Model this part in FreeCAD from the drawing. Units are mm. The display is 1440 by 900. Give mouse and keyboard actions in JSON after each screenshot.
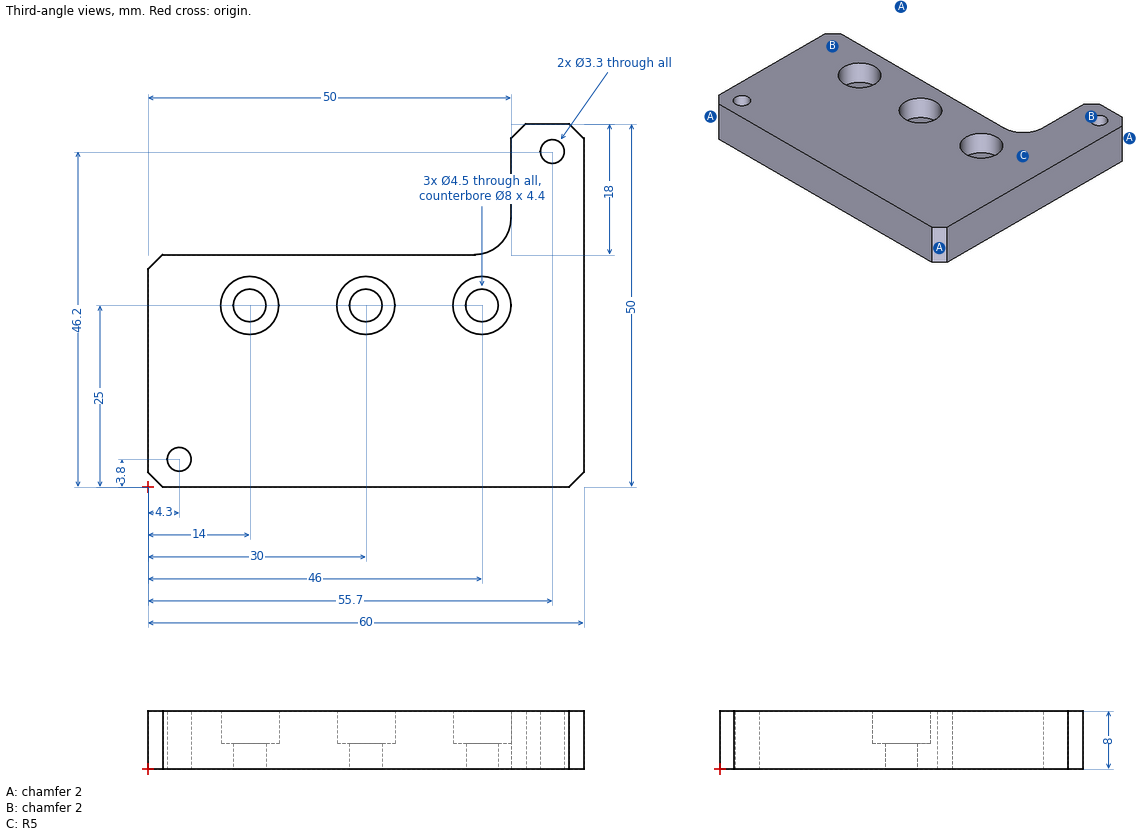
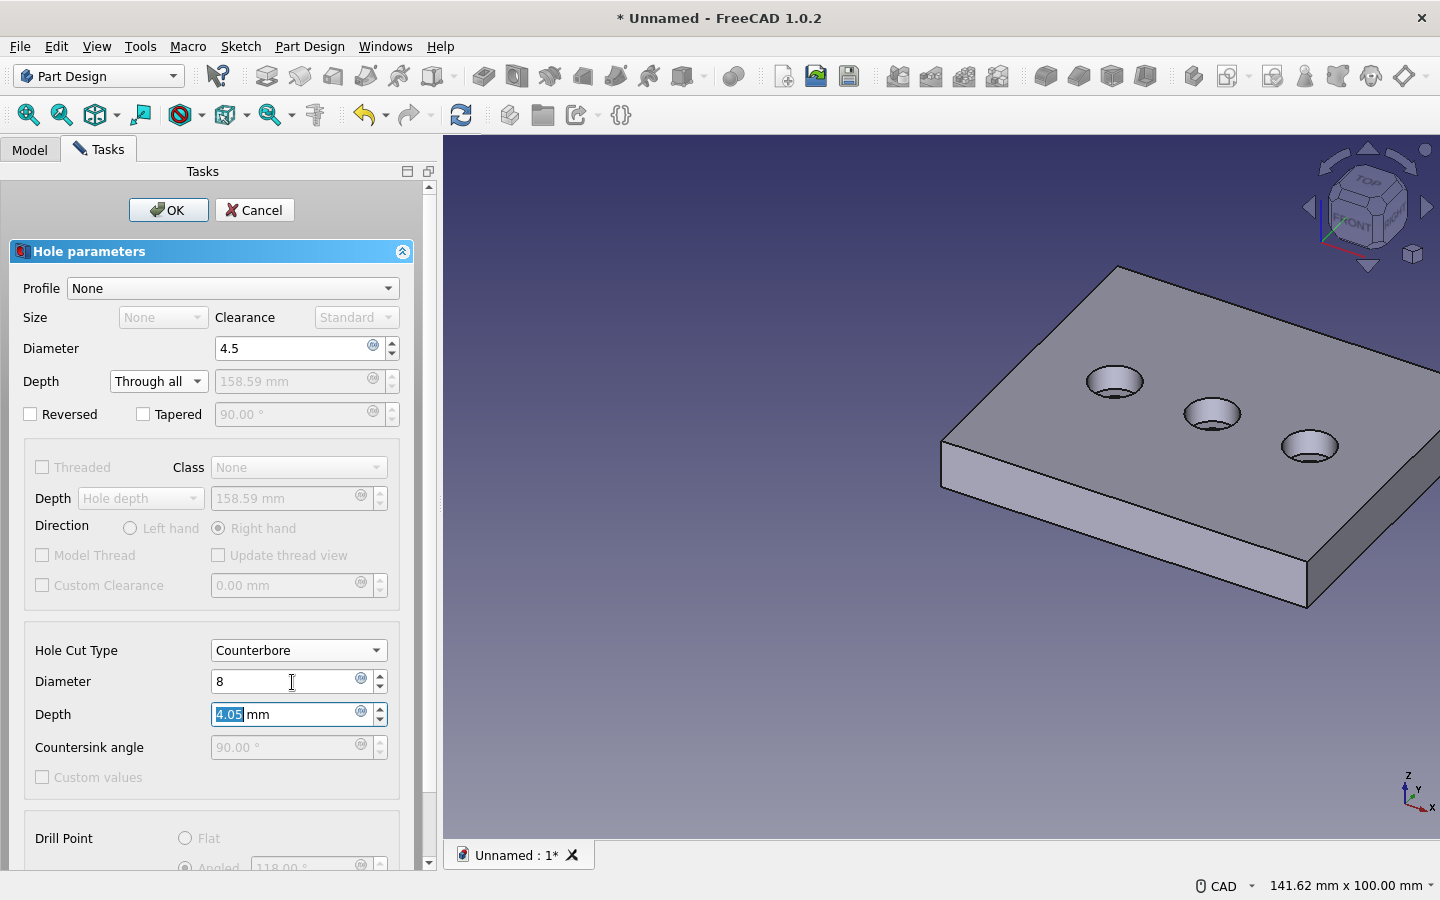
{"action": "type", "text": "4.4"}
{"action": "key", "text": "Tab"}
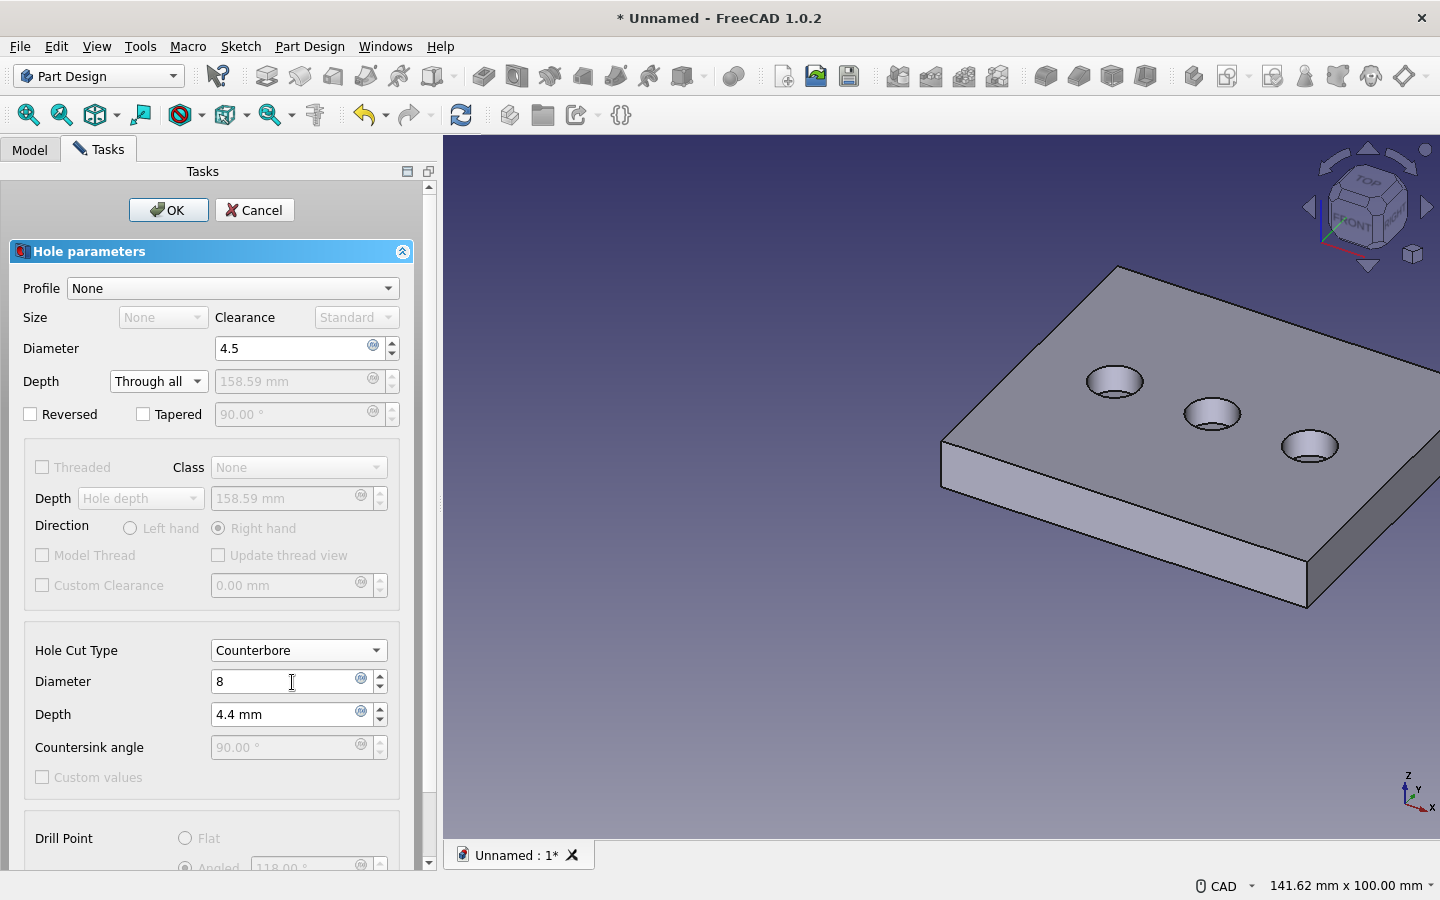
{"action": "left_click", "coordinate": [169, 210]}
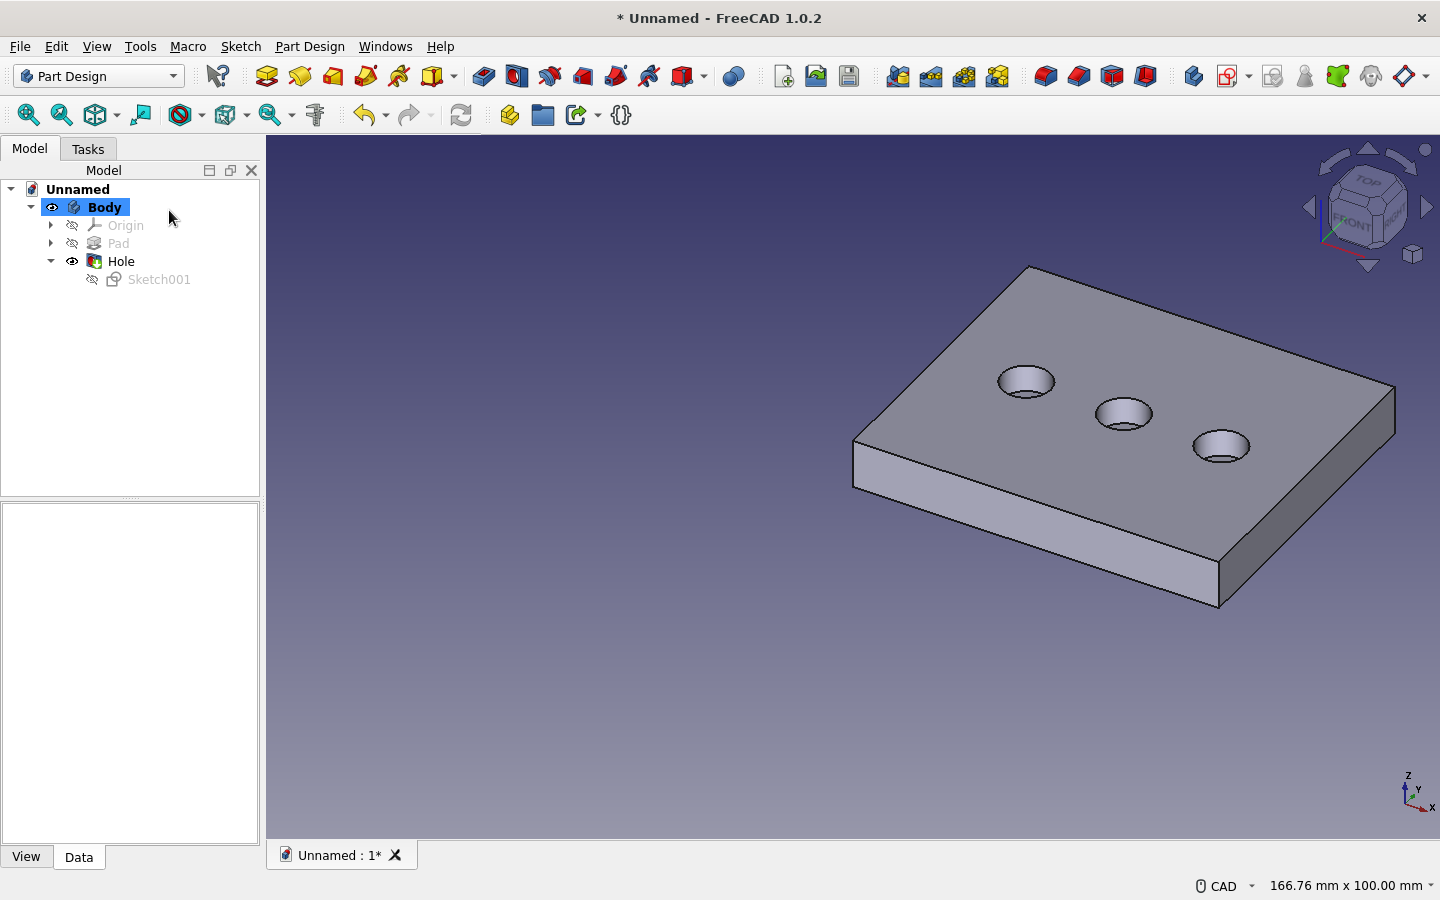
{"action": "left_click", "coordinate": [1226, 380]}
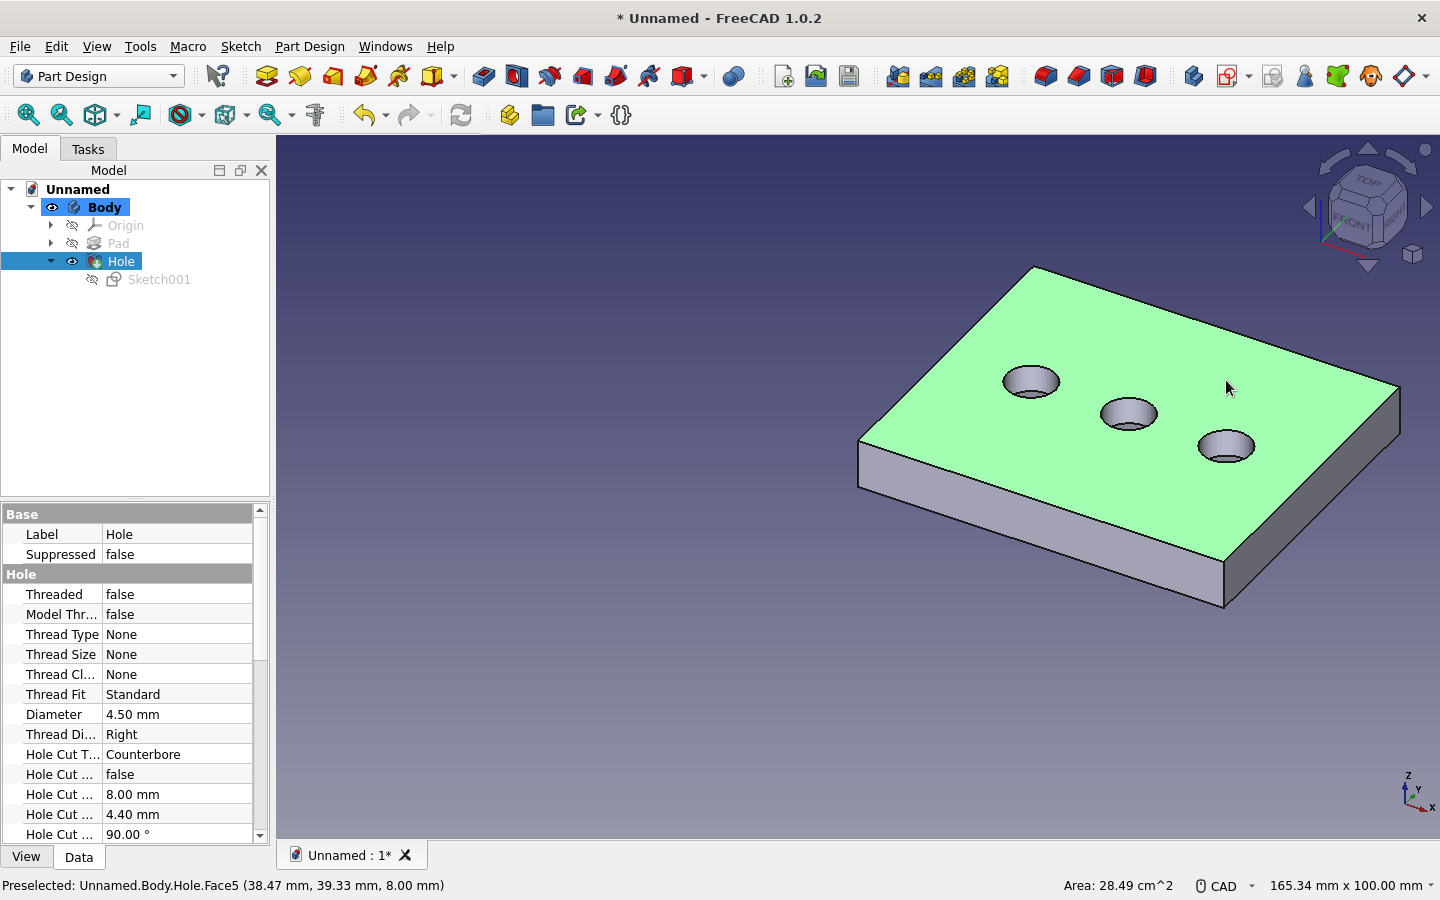
{"action": "left_click", "coordinate": [1226, 76]}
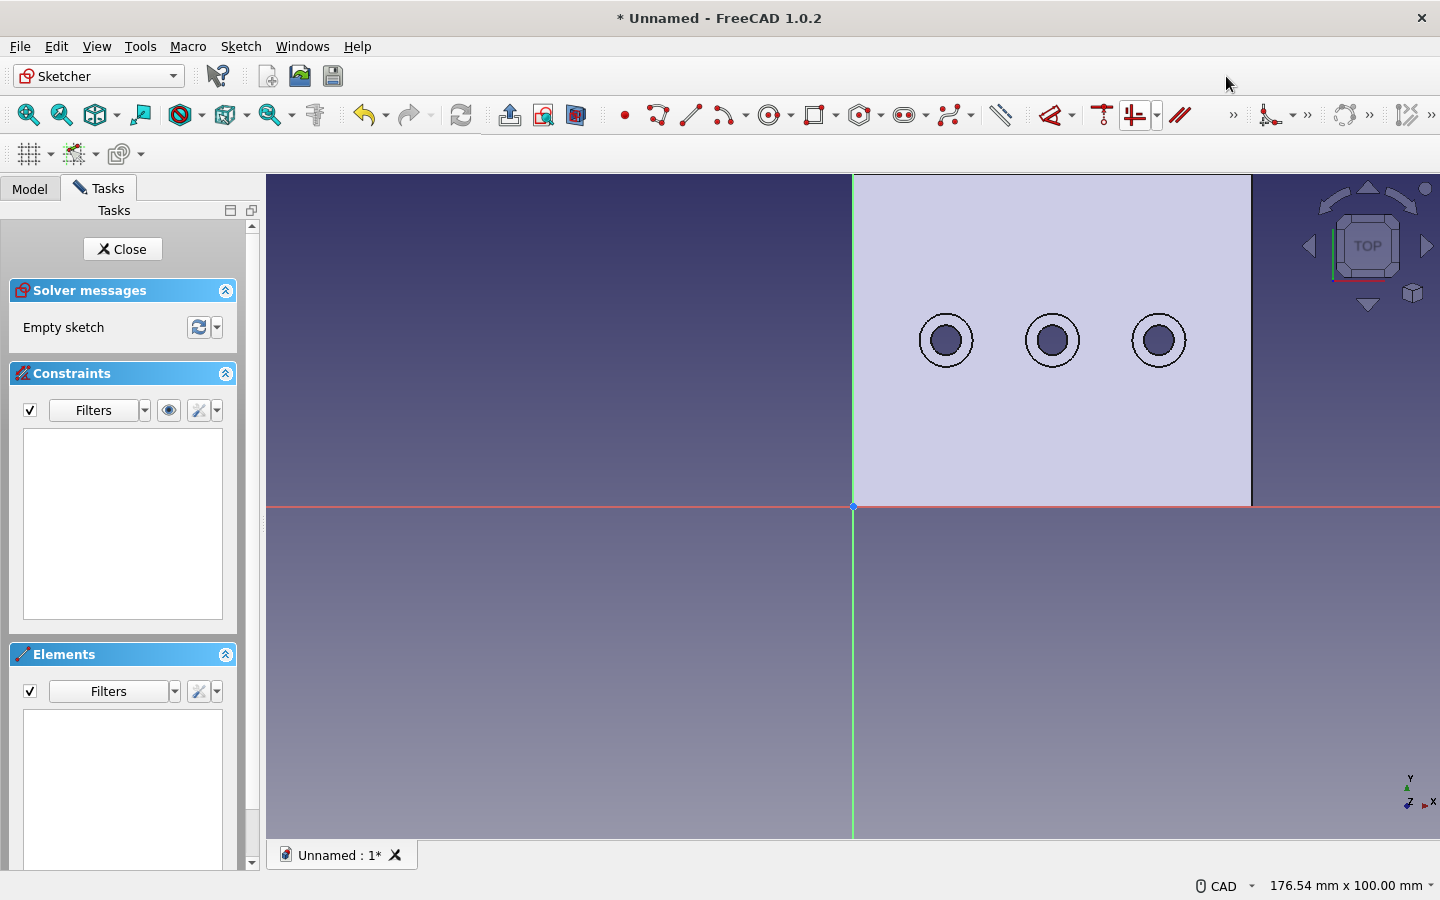
{"action": "scroll", "coordinate": [294, 811], "scroll_direction": "down", "scroll_amount": 1}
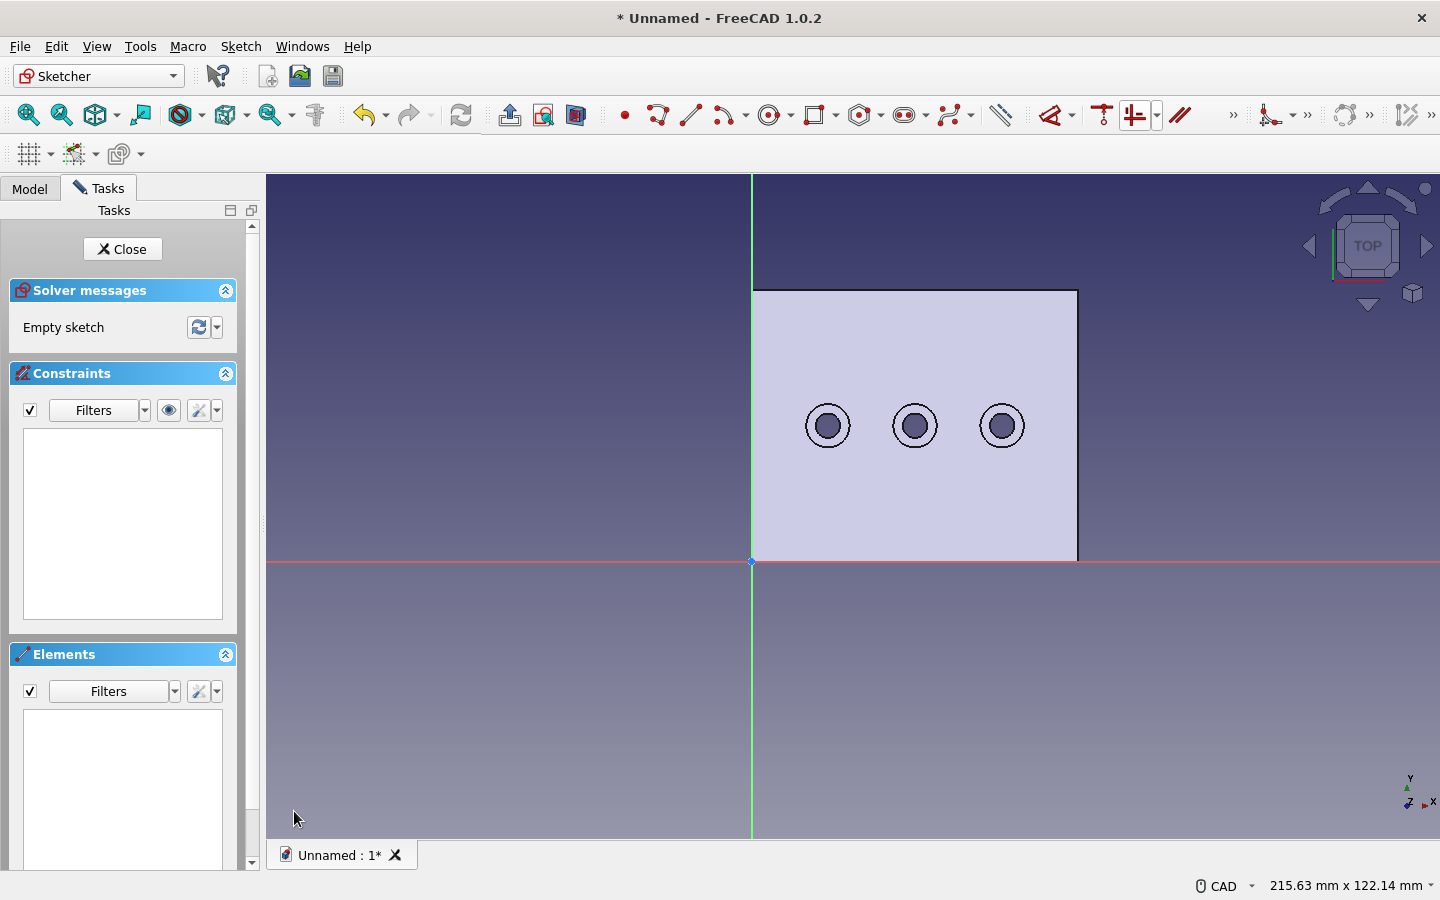
{"action": "scroll", "coordinate": [1058, 341], "scroll_direction": "up", "scroll_amount": 3}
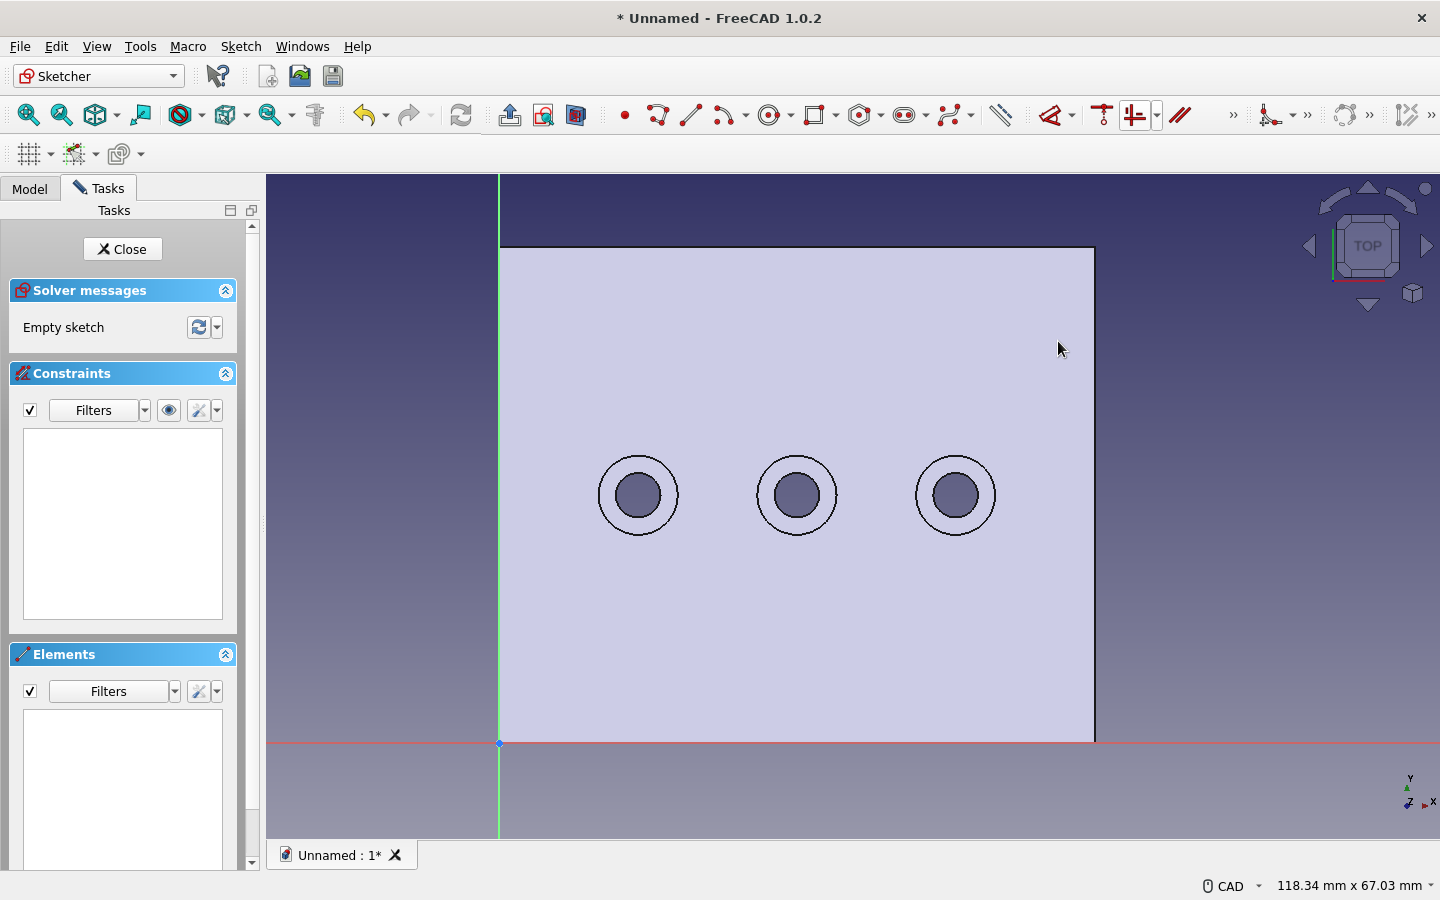
{"action": "left_click", "coordinate": [768, 116]}